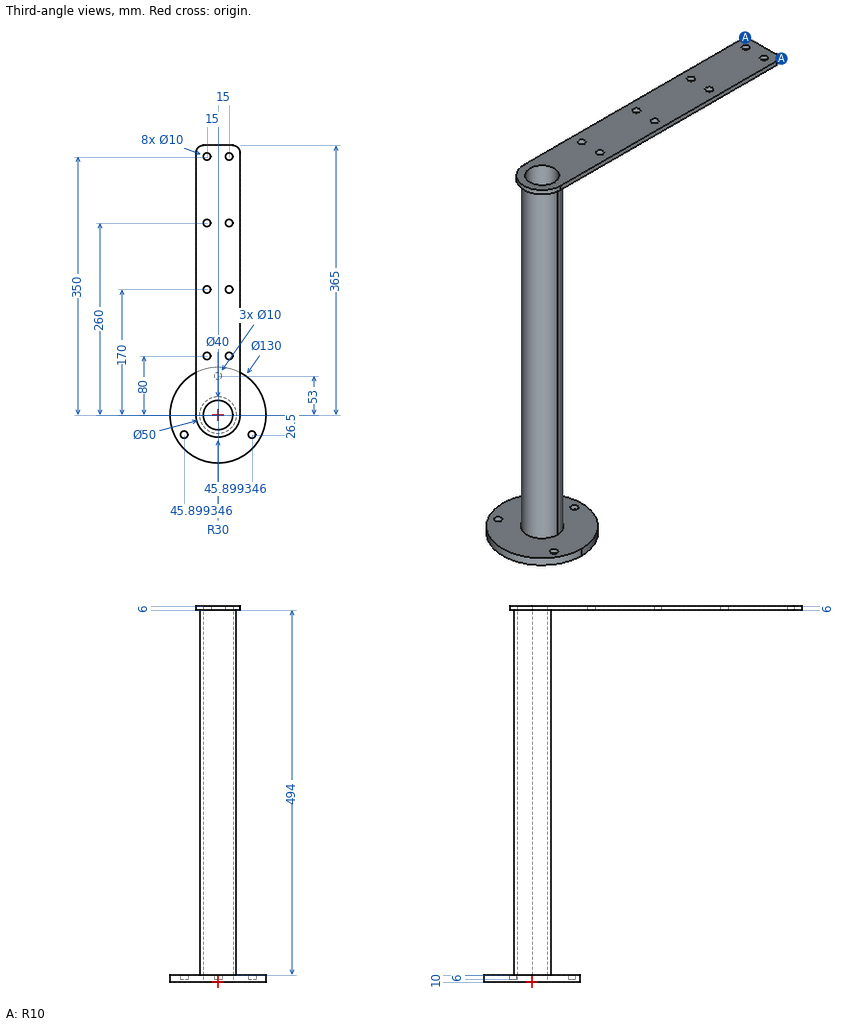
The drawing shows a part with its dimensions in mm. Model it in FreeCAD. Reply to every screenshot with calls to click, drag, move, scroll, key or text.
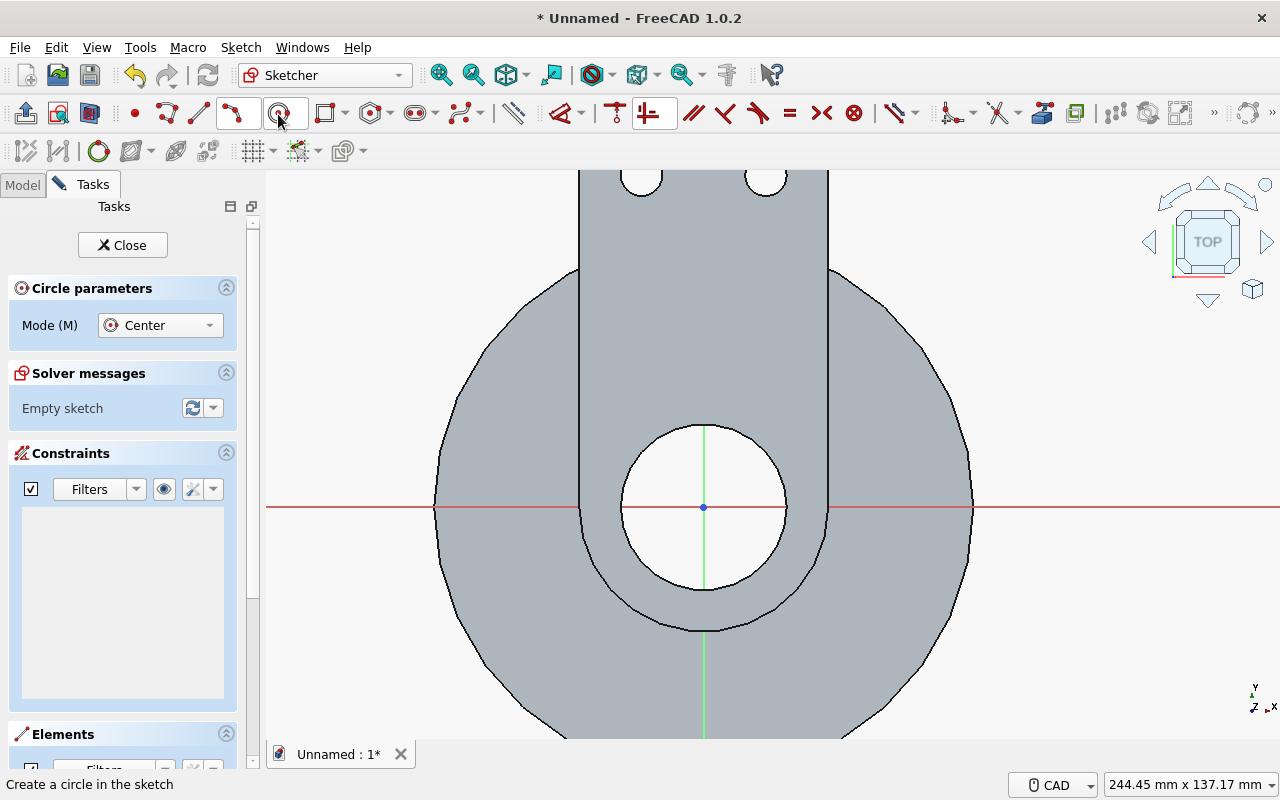
click(704, 287)
move(718, 273)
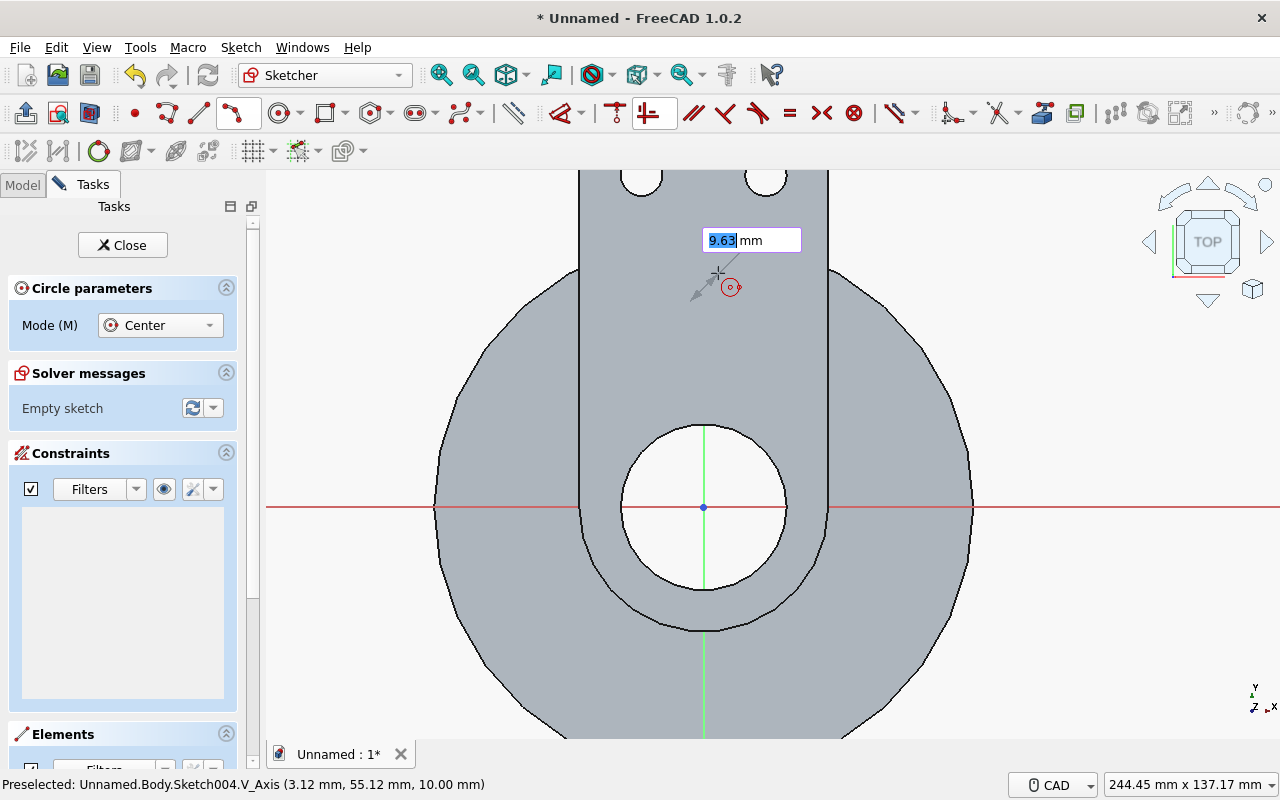
text(10)
key(Return)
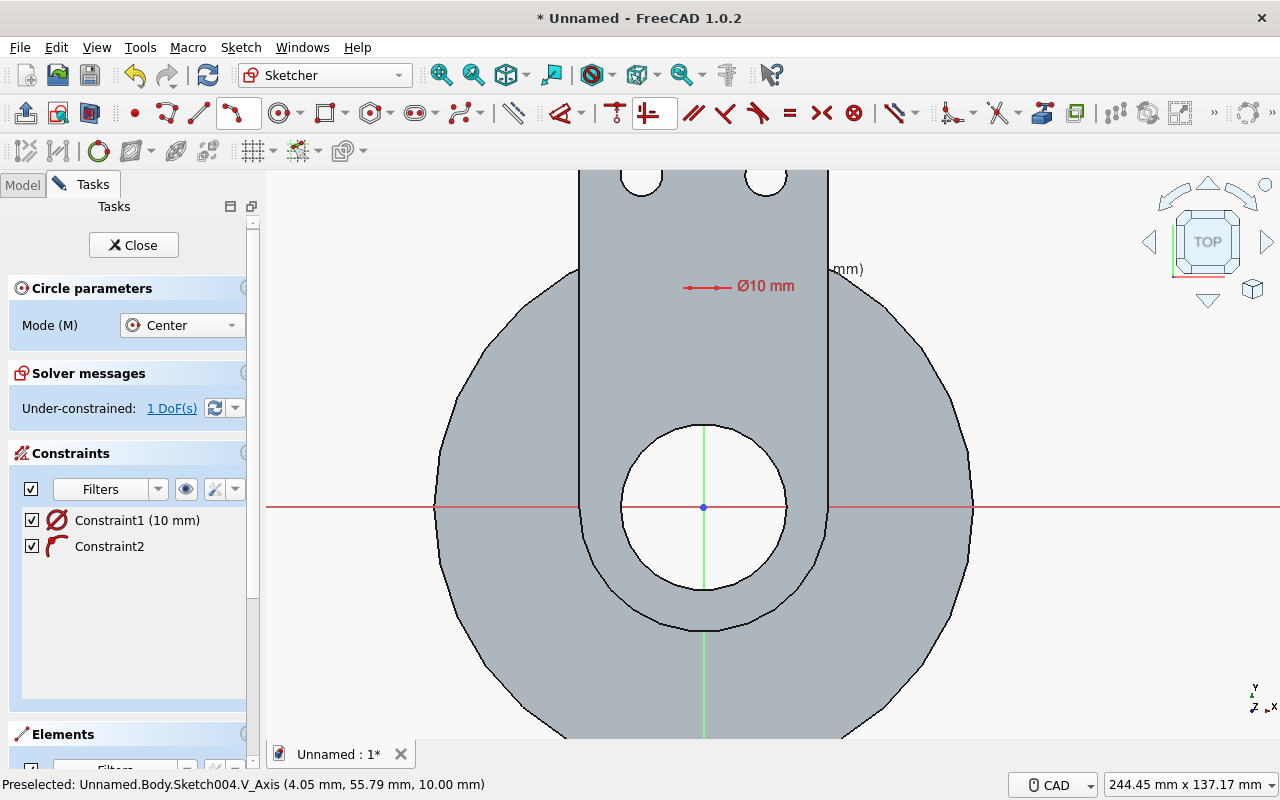
click(894, 617)
move(909, 602)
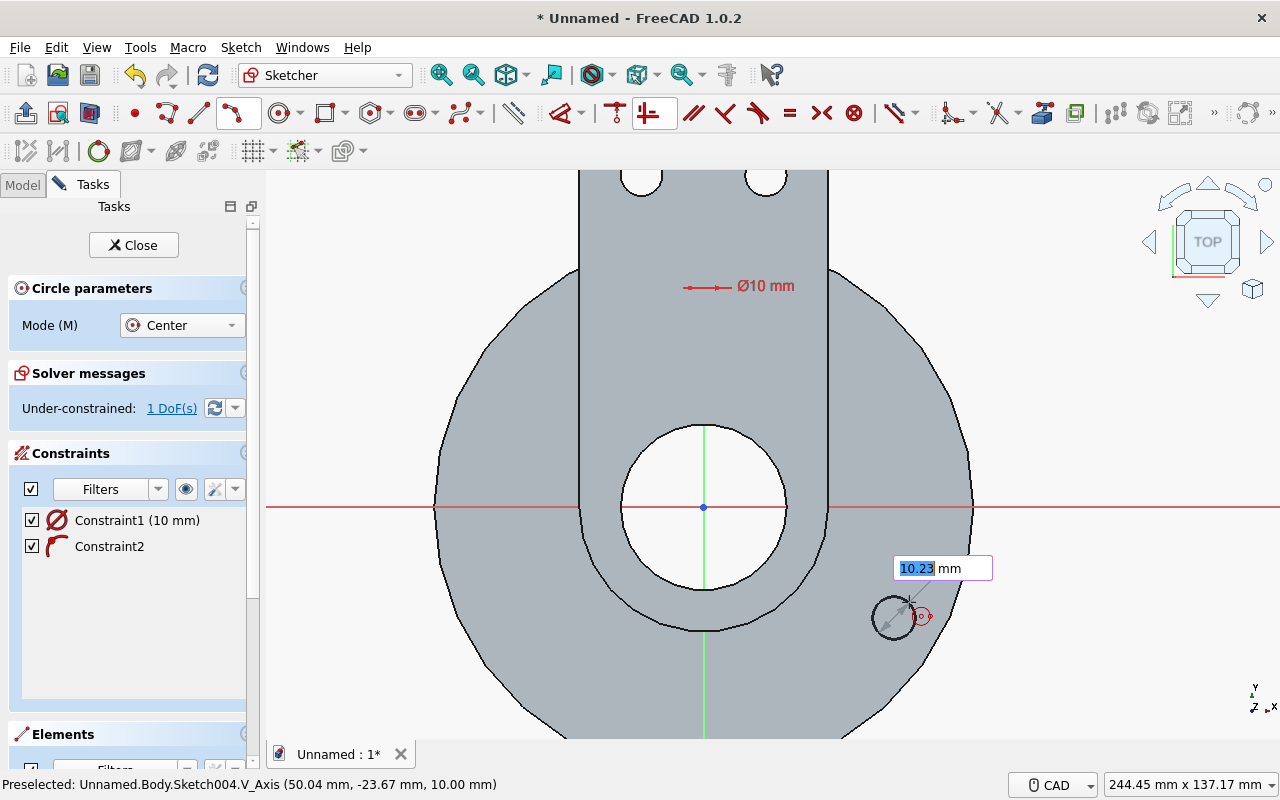
text(10)
key(Return)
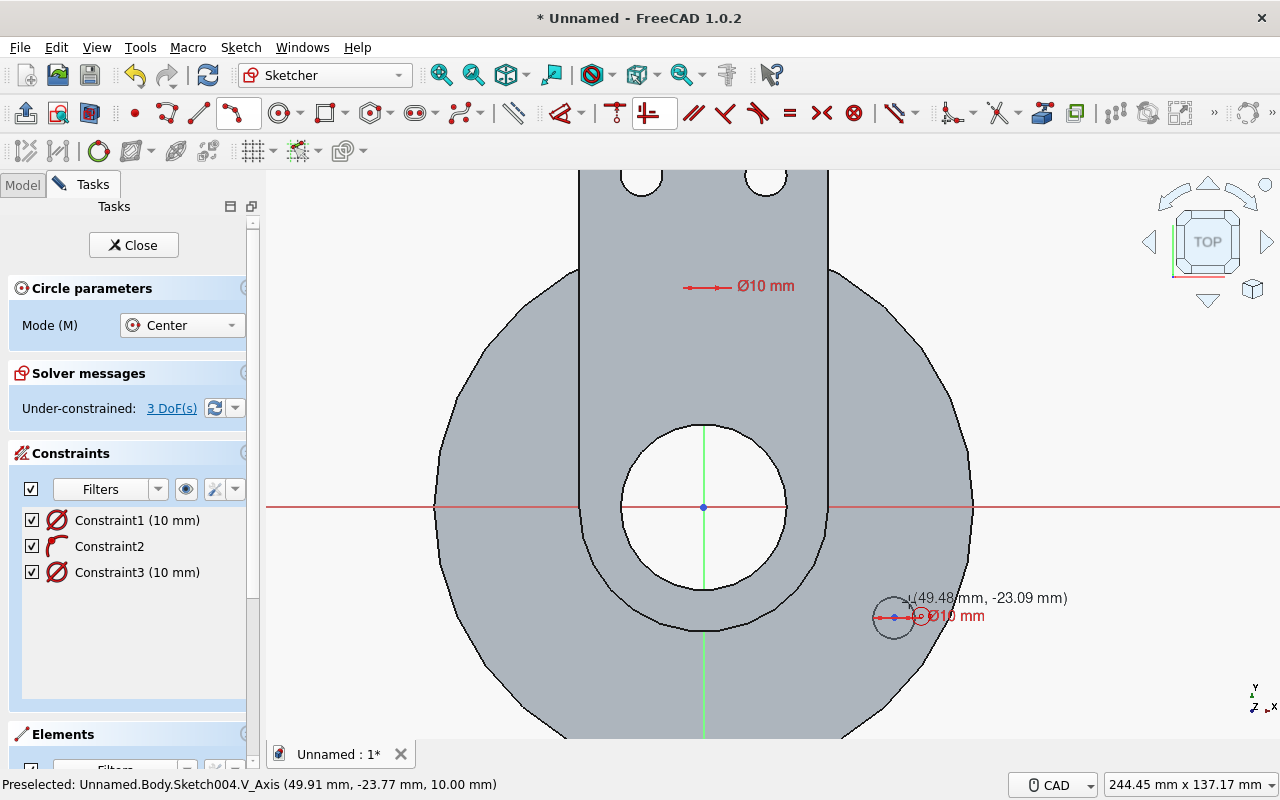
click(513, 617)
move(528, 602)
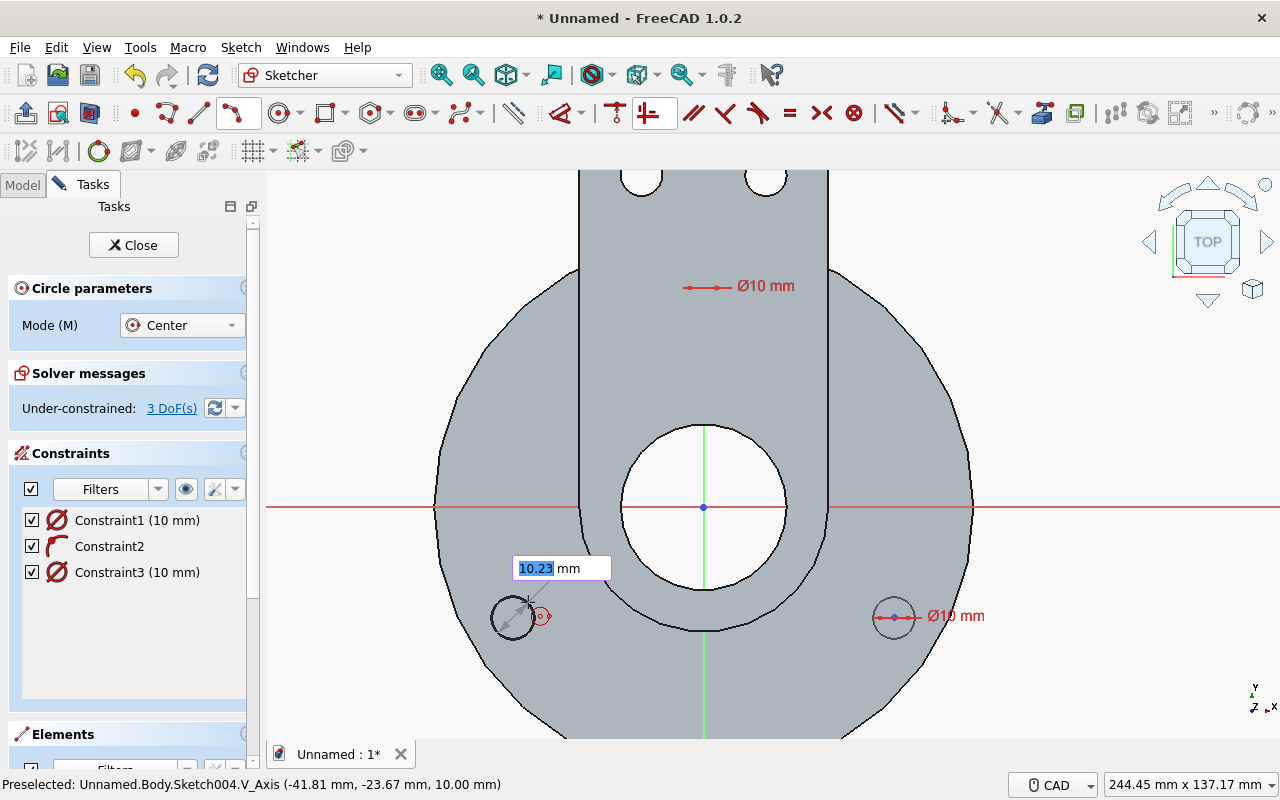
text(10)
key(Return)
key(Escape)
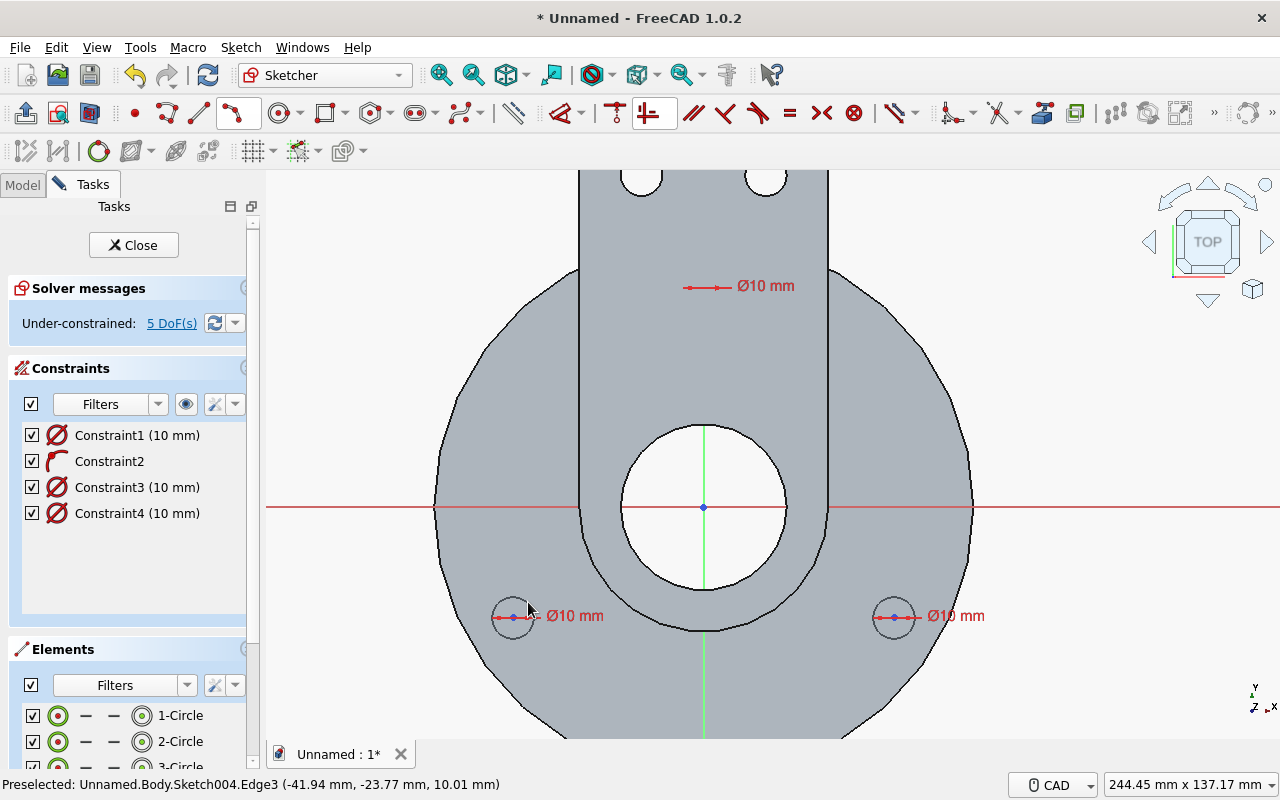
click(894, 618)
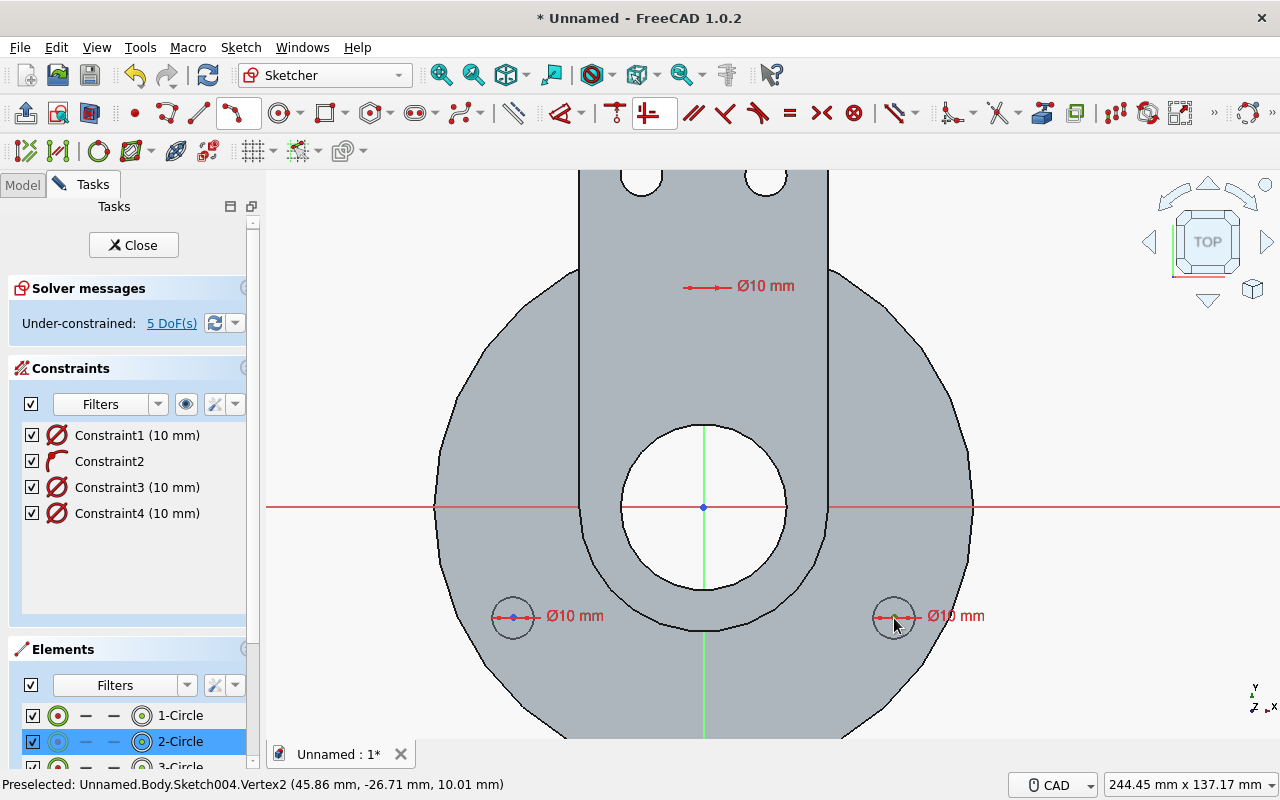
click(513, 618)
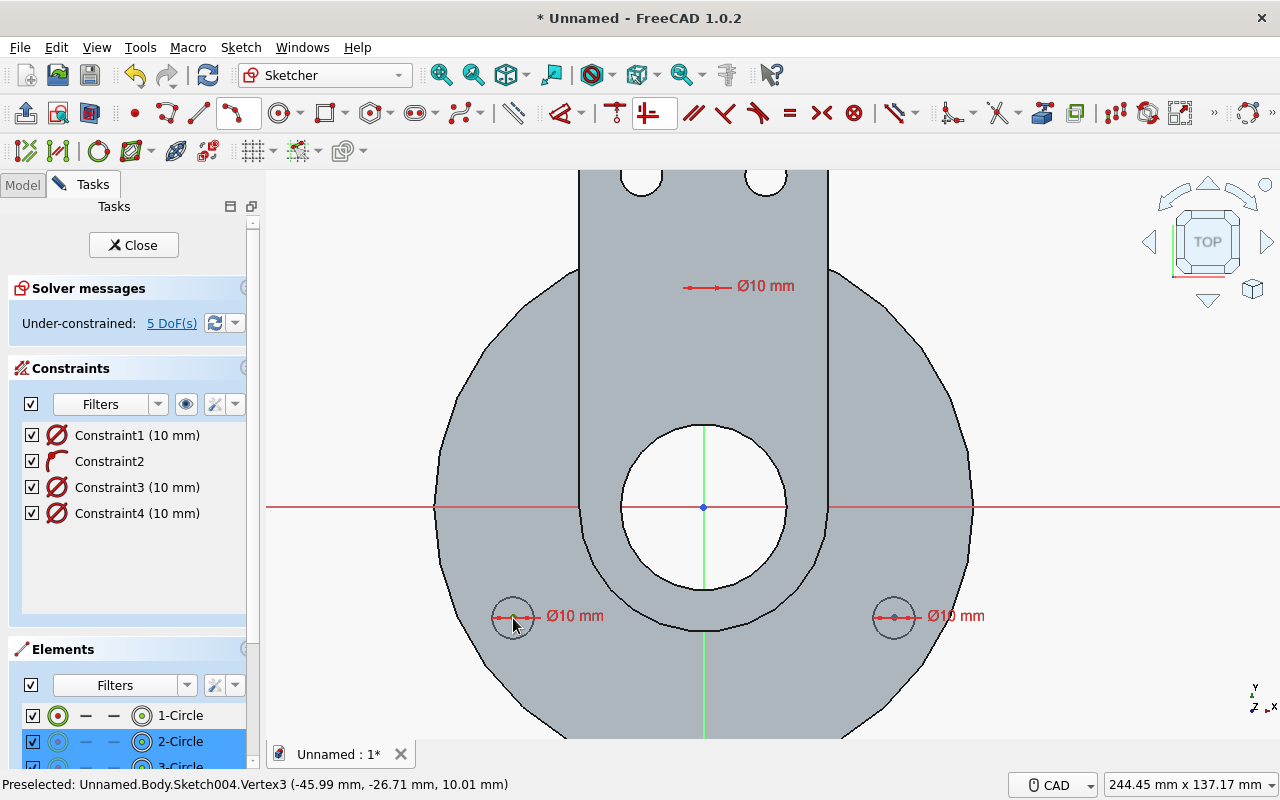
click(672, 114)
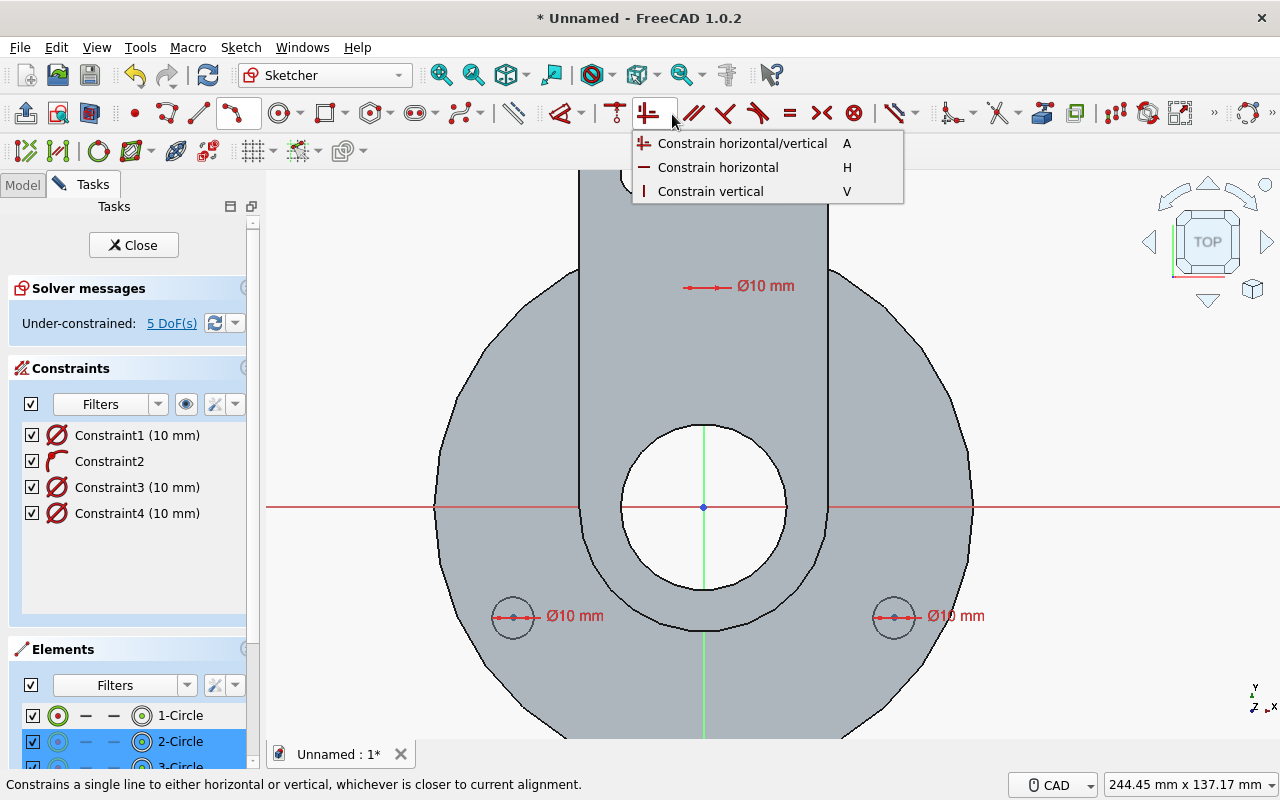
click(768, 167)